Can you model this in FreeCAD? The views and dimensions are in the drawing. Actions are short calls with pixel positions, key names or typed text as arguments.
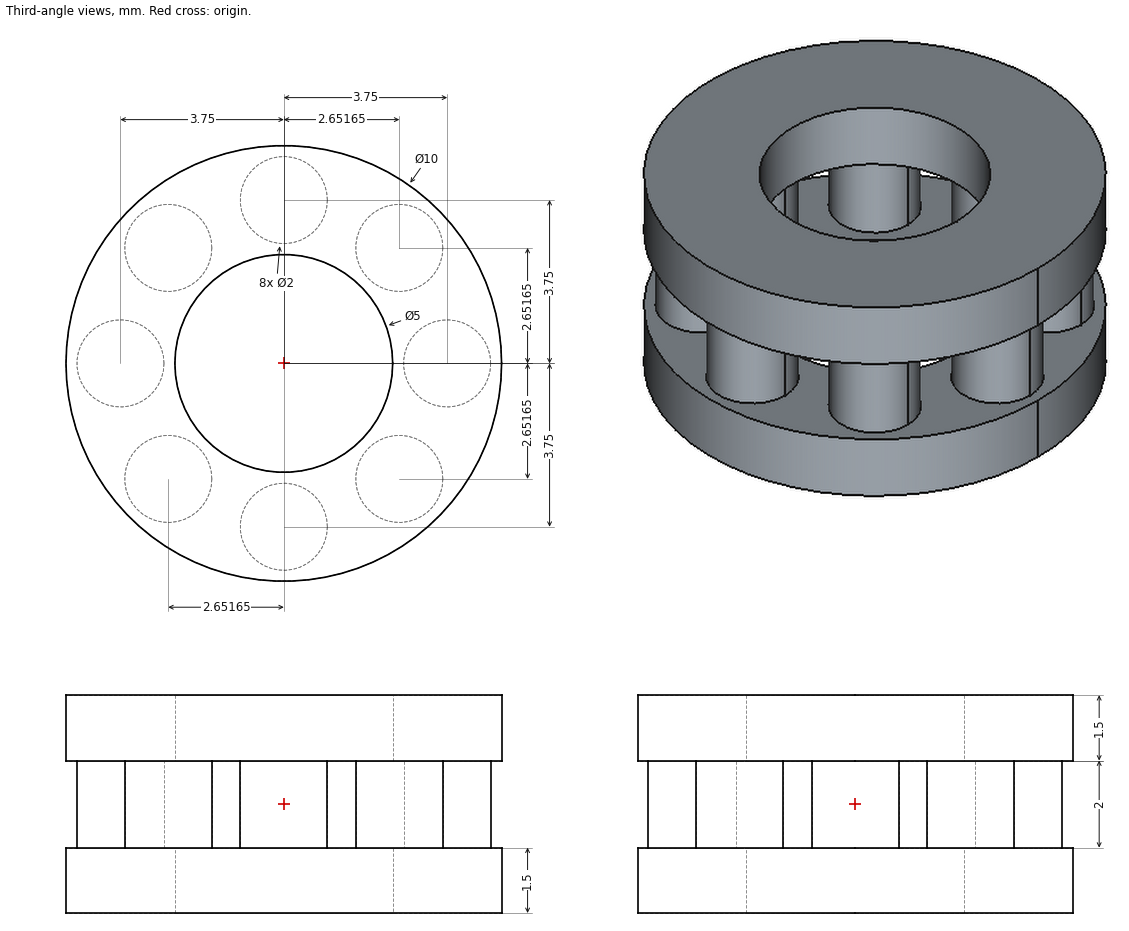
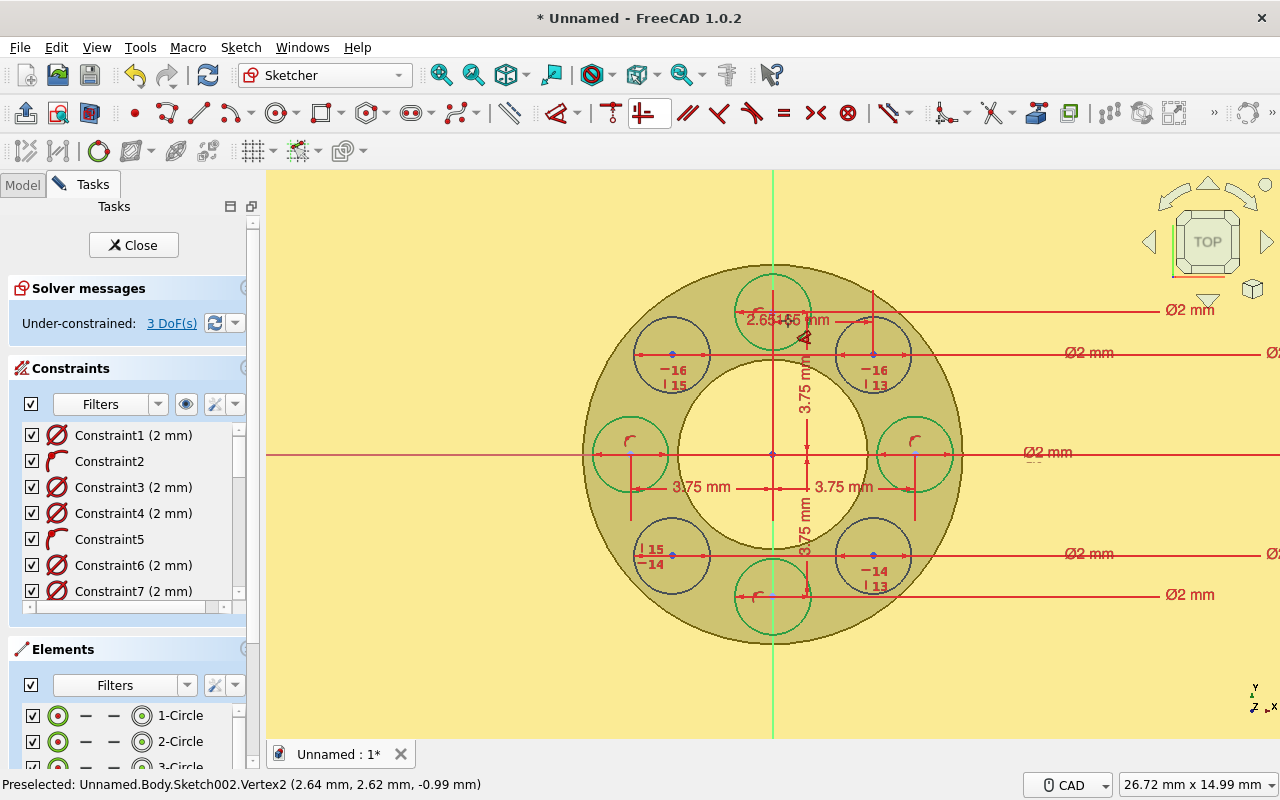
click(873, 355)
click(907, 440)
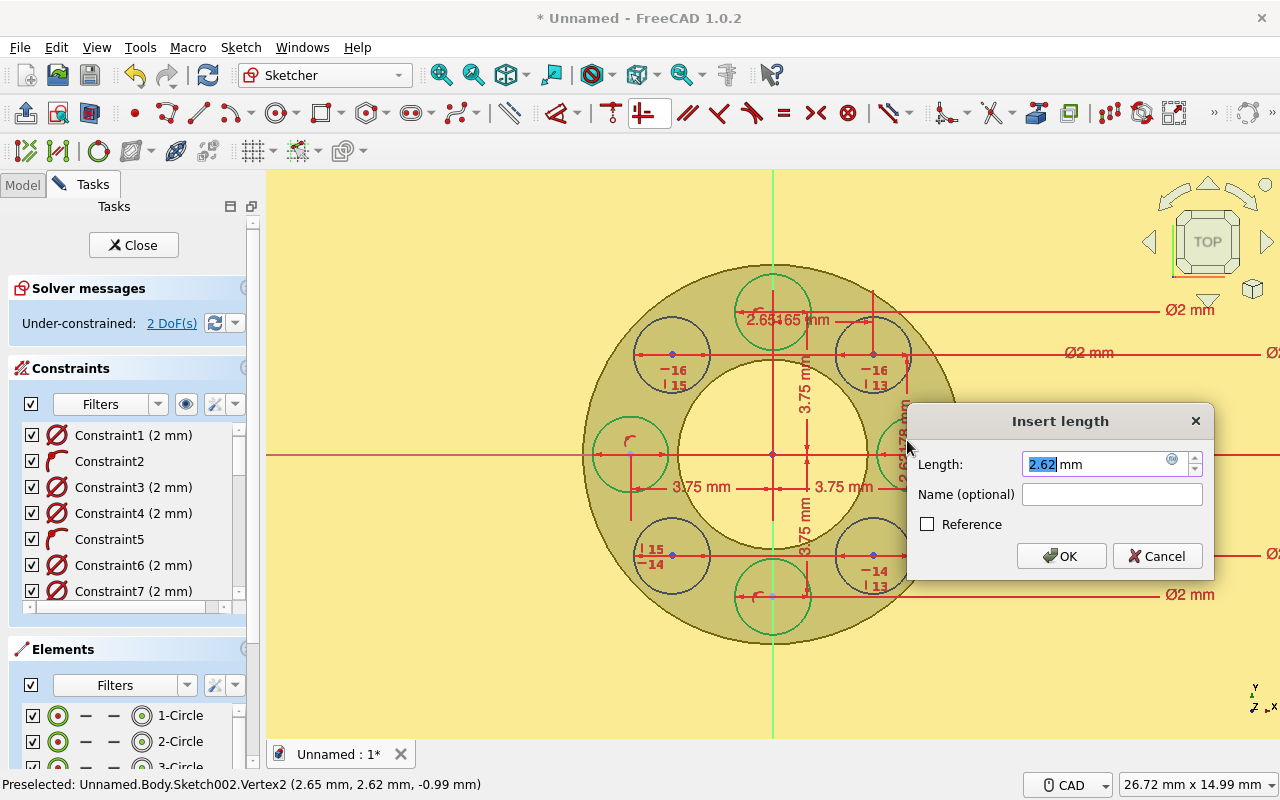
text(2.65165)
key(Return)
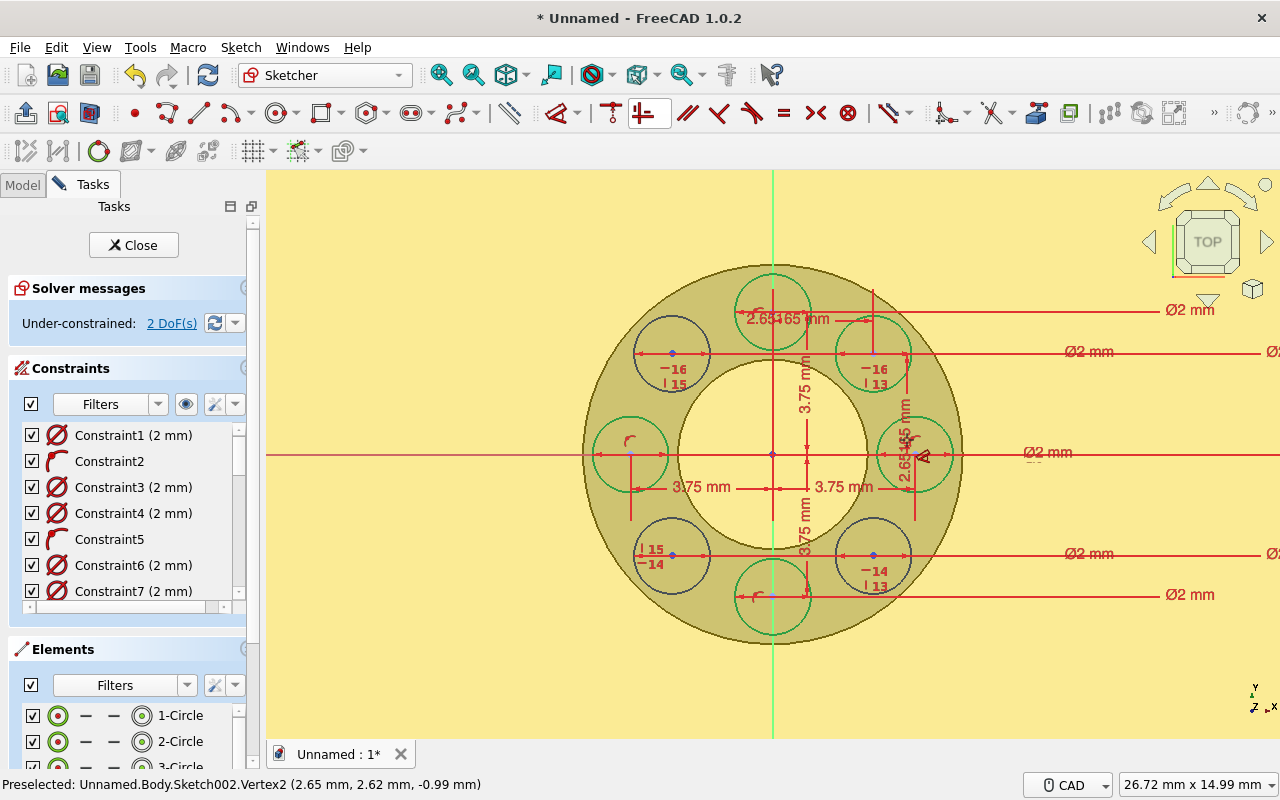
click(873, 556)
click(931, 505)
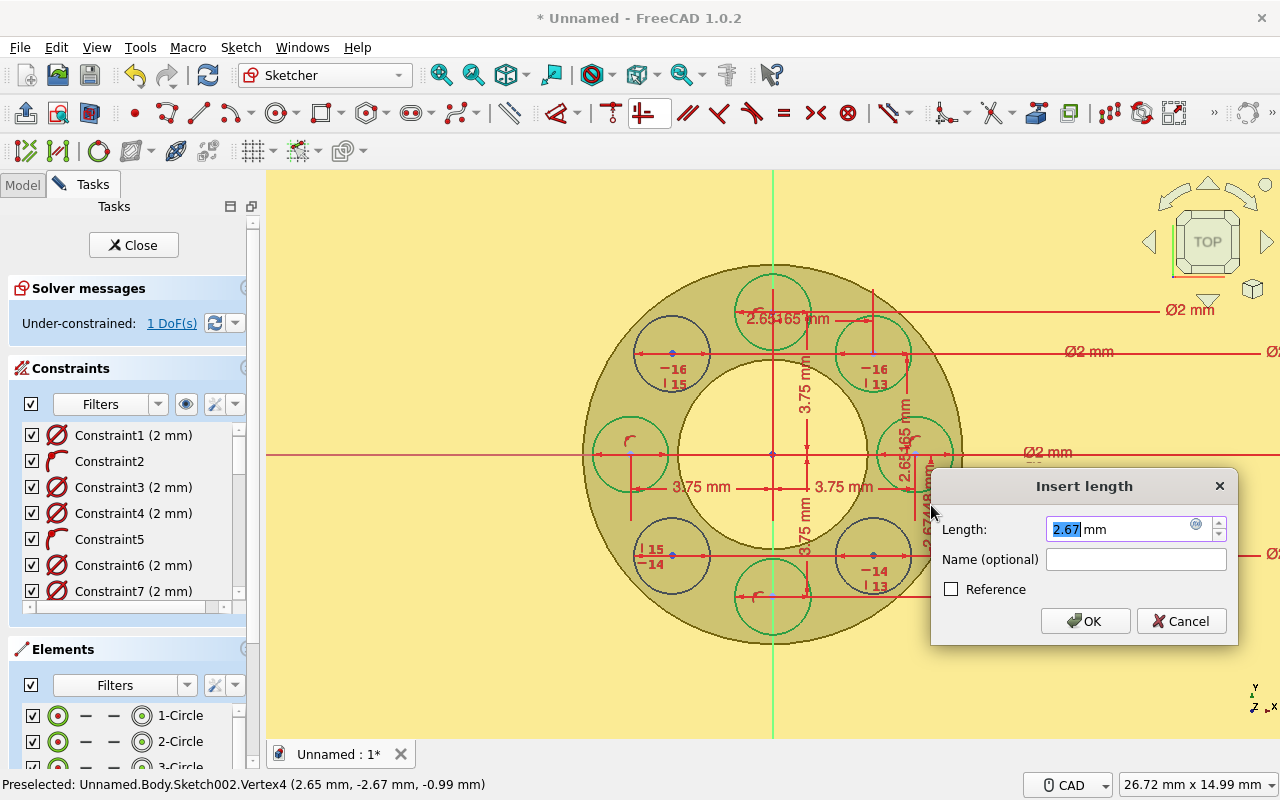
text(2.65165)
key(Return)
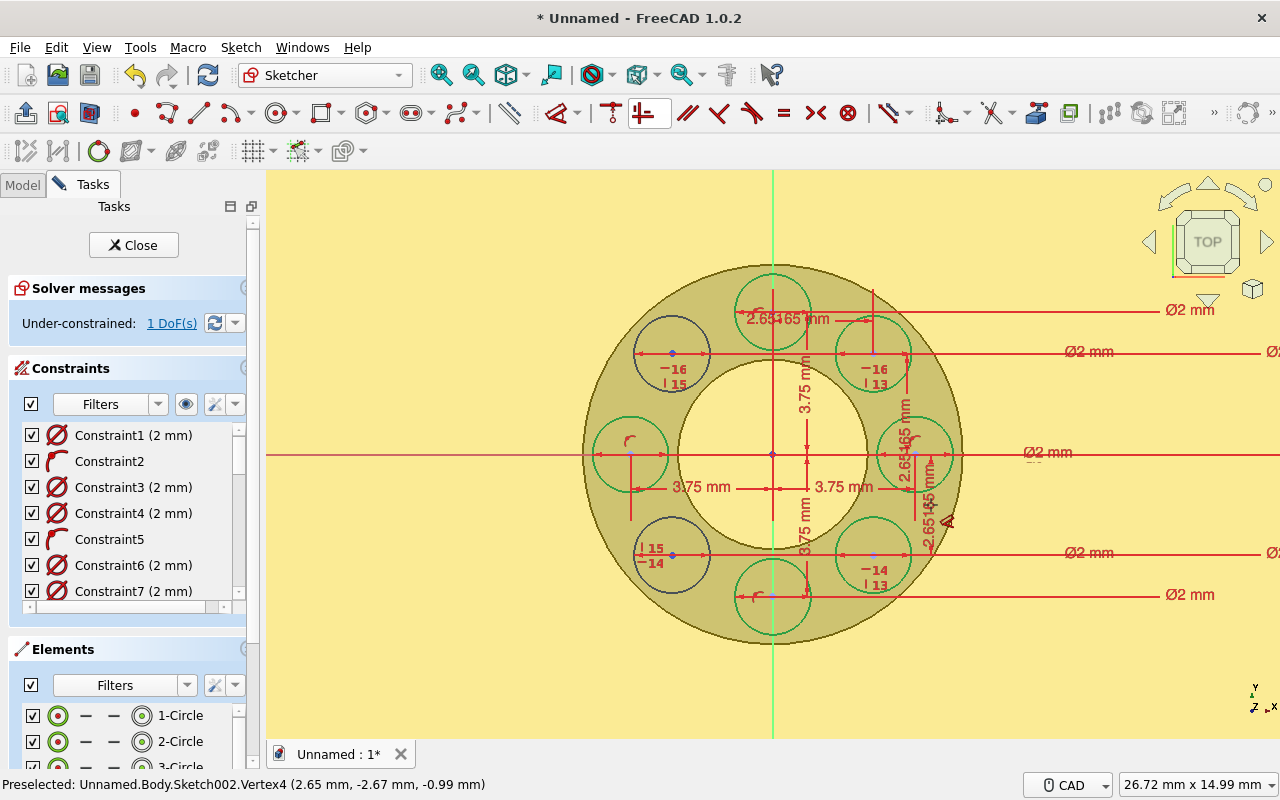
click(672, 555)
click(722, 589)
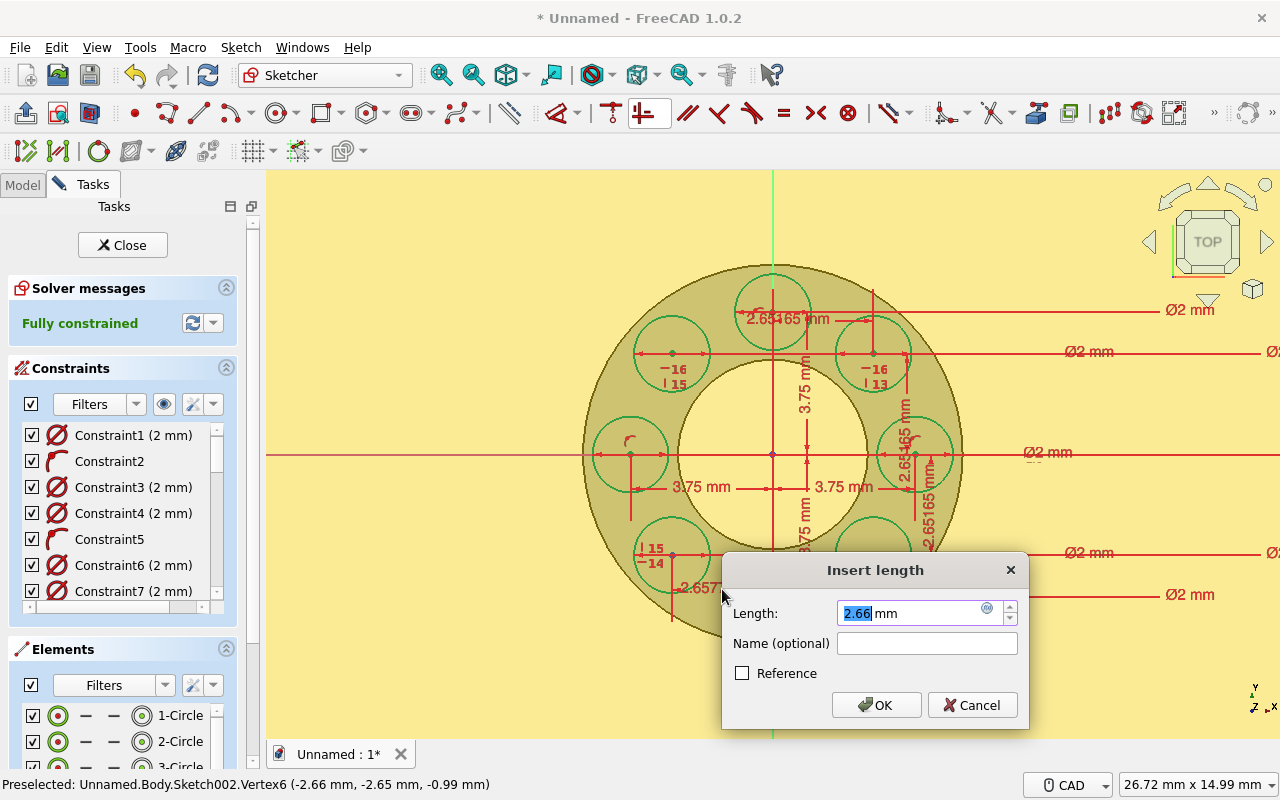
text(2.65165)
key(Return)
key(Escape)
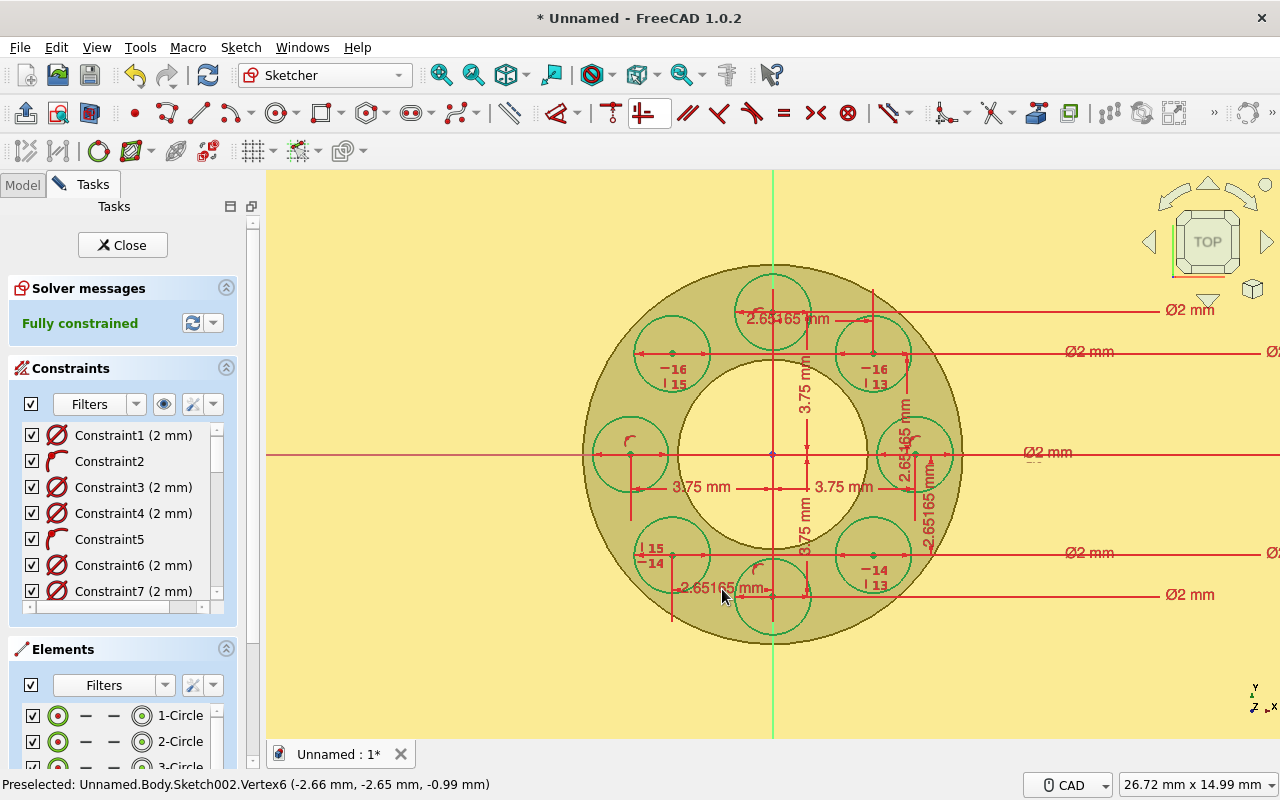
click(123, 245)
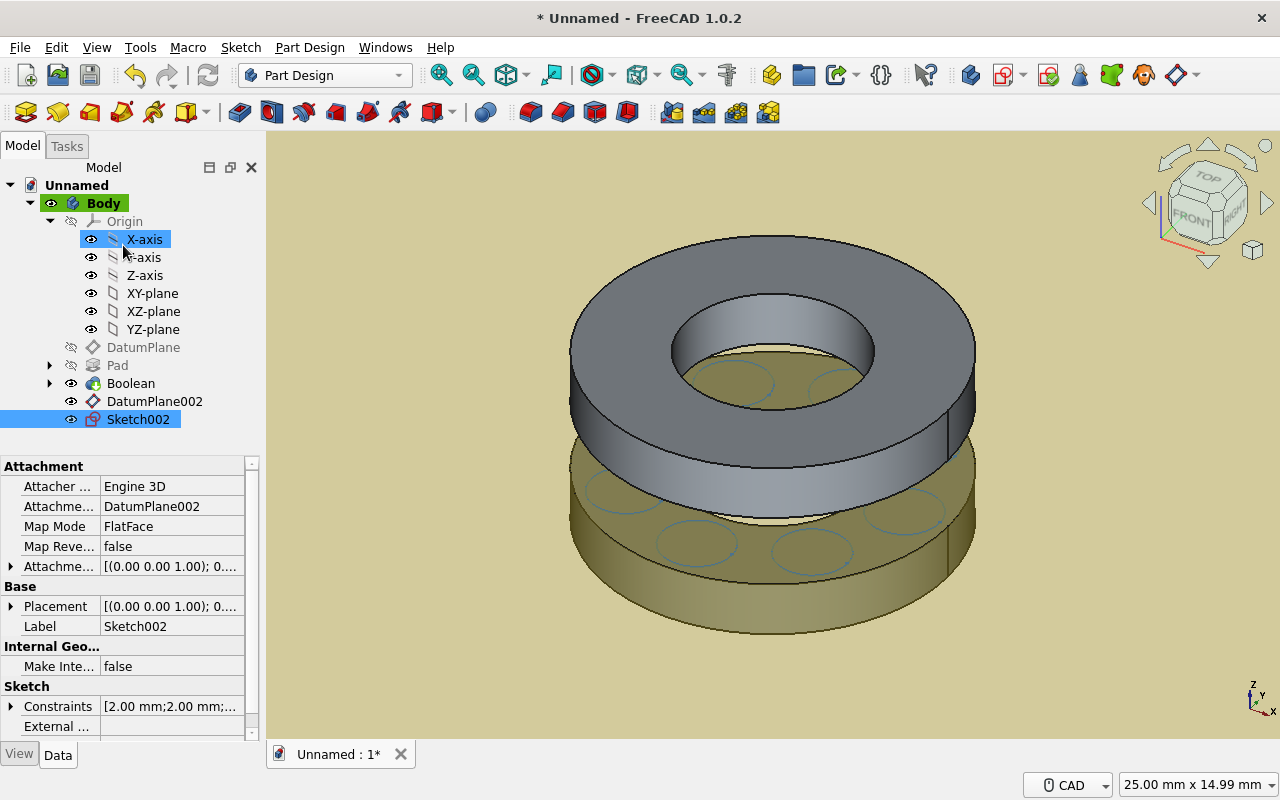
click(26, 112)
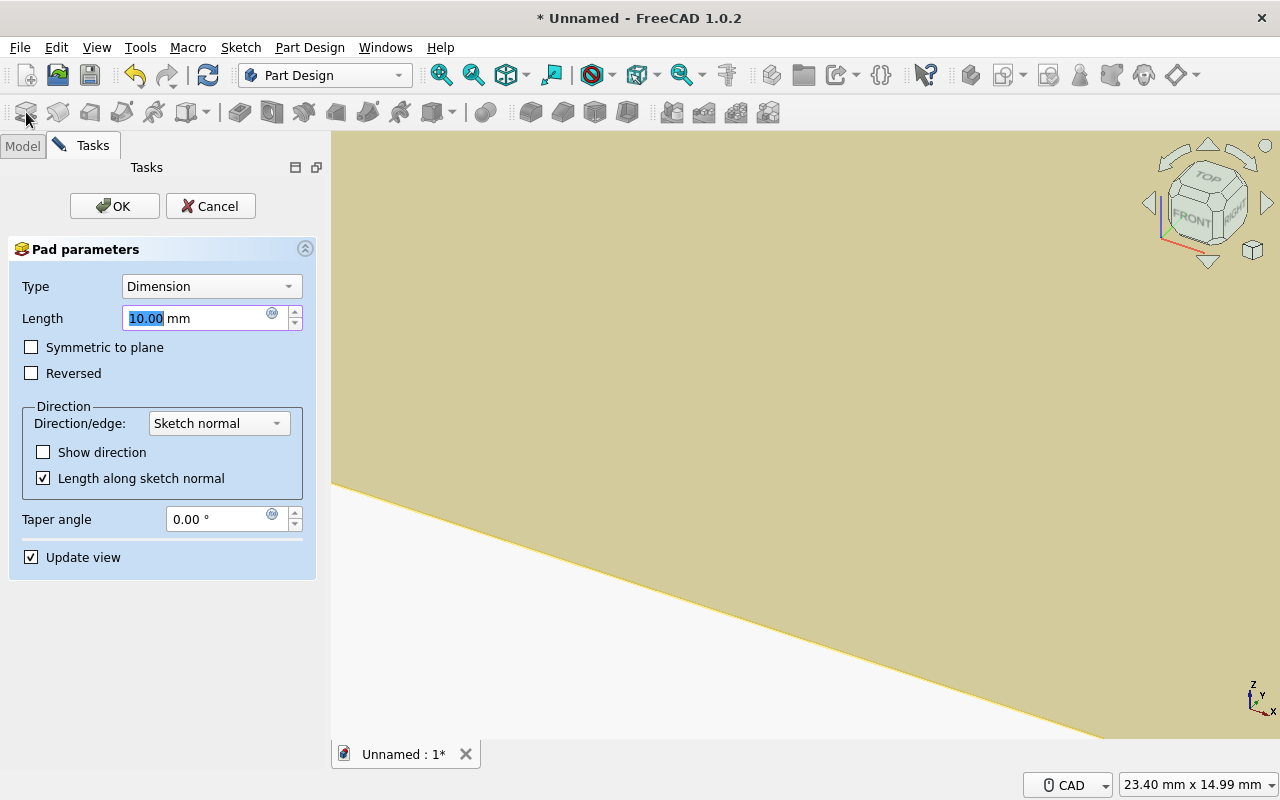
text(2)
key(Tab)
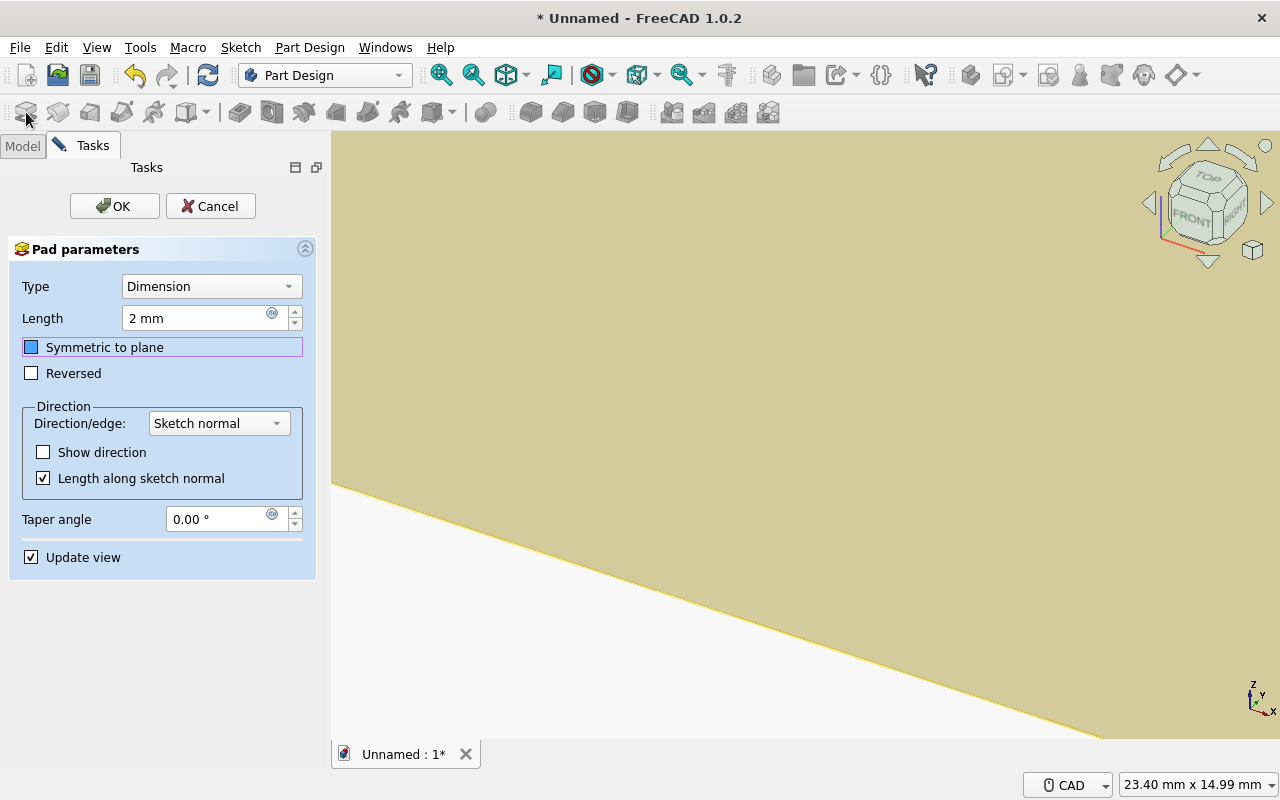
click(115, 206)